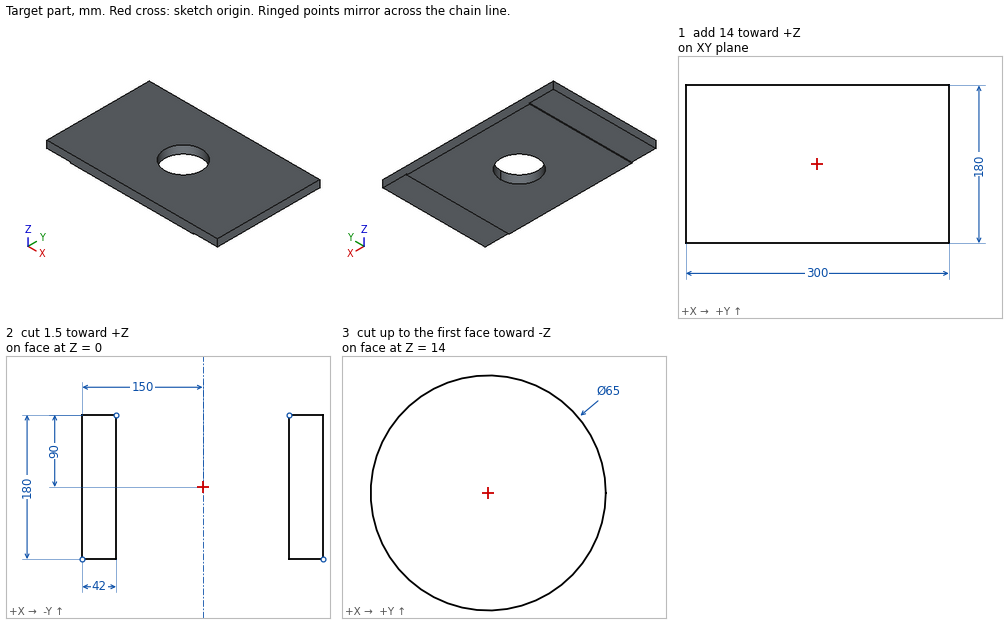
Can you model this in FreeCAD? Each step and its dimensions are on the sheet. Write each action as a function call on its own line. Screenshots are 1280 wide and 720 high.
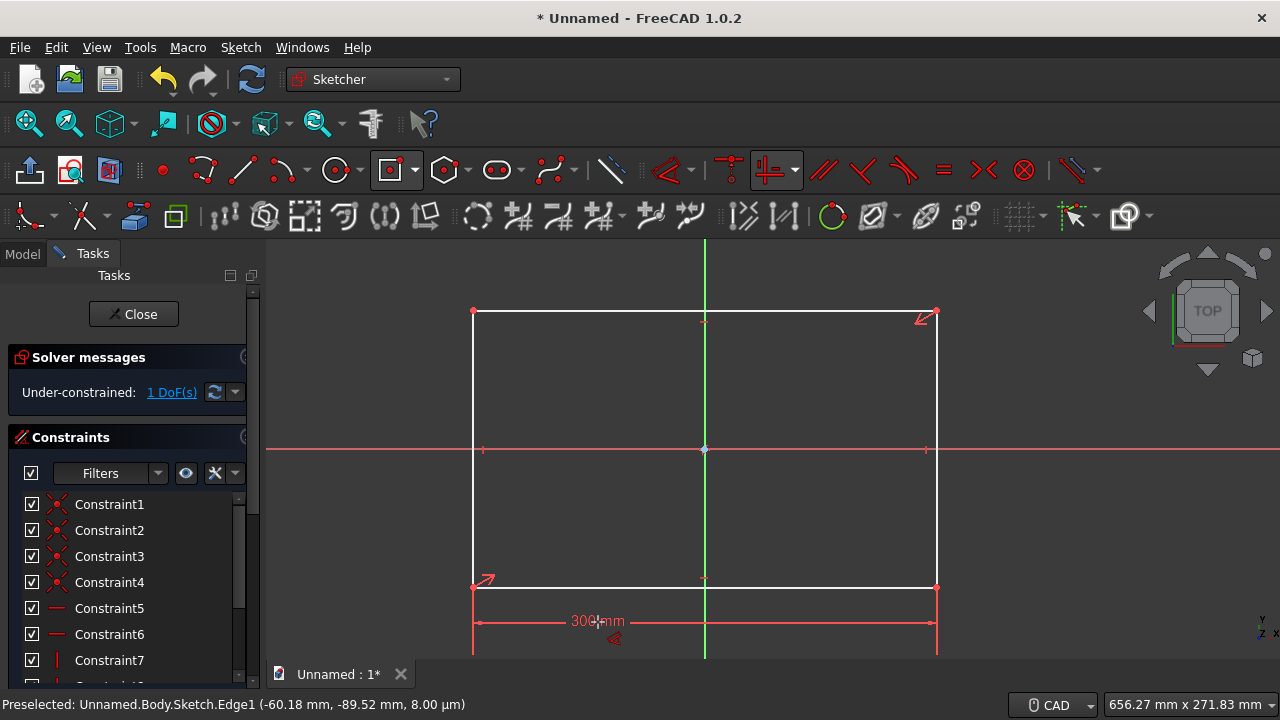
click(937, 505)
click(971, 386)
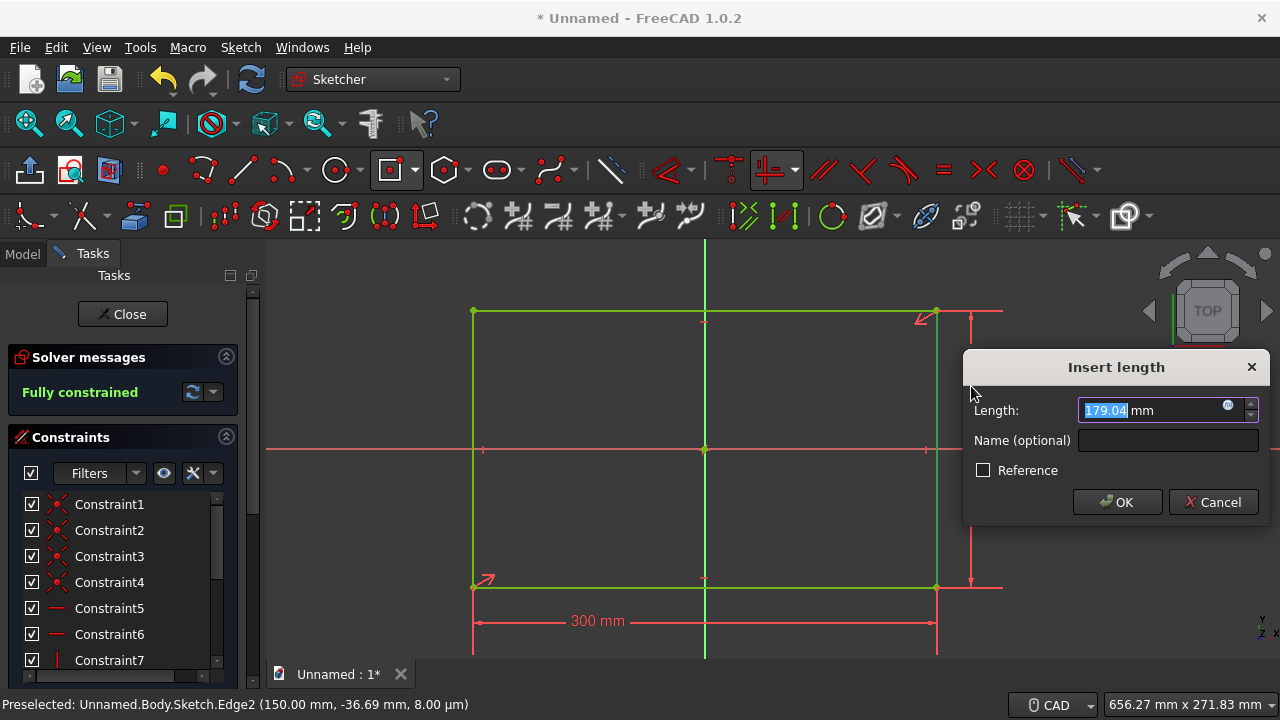
text(180)
key(Return)
key(Escape)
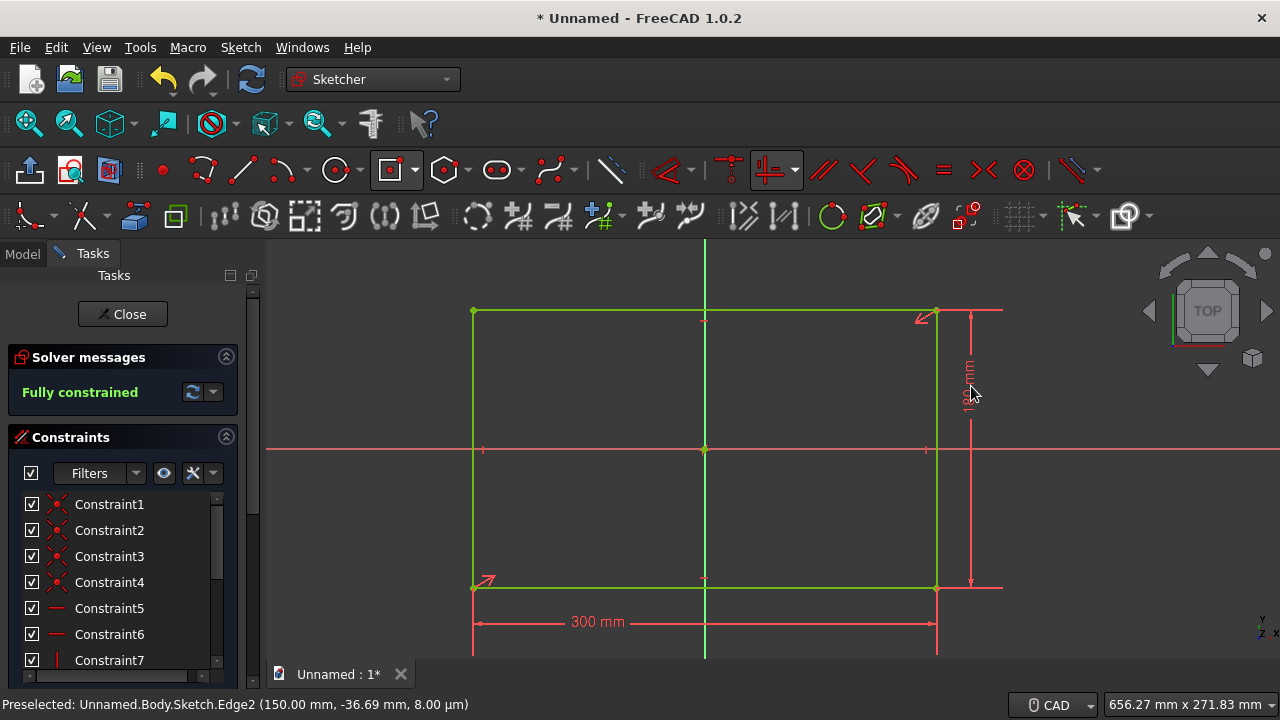
click(123, 314)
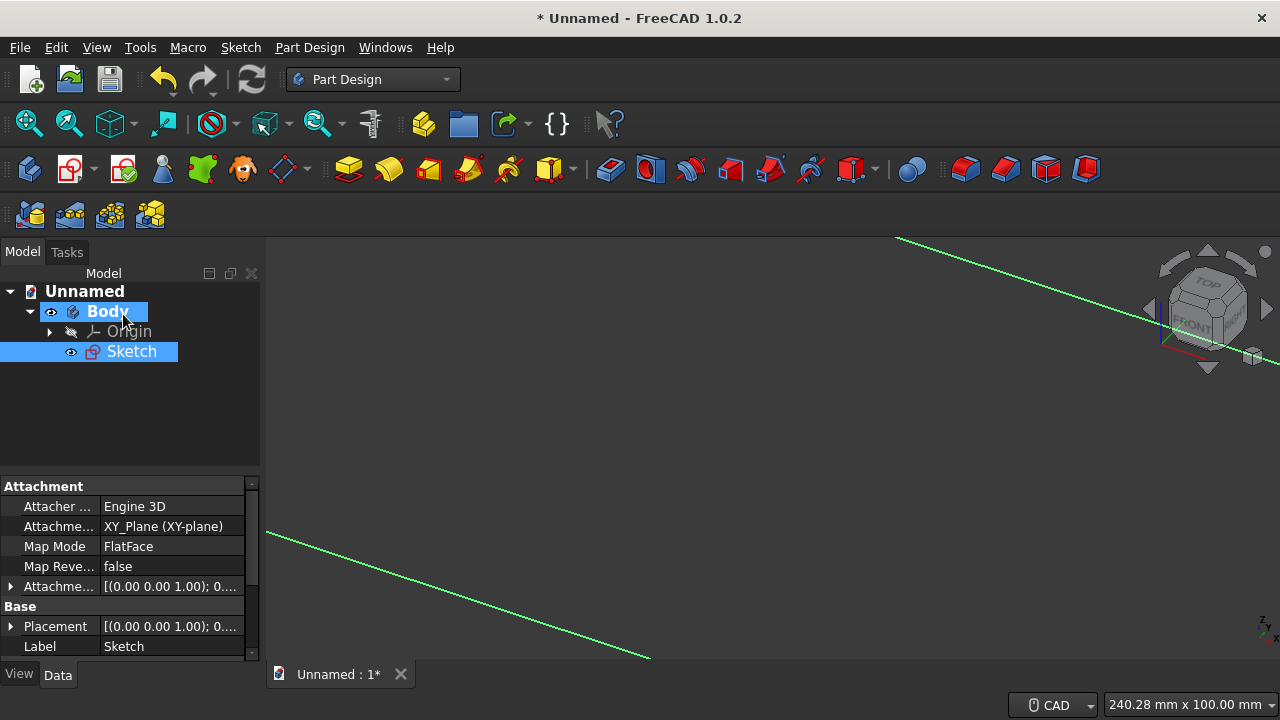
click(350, 170)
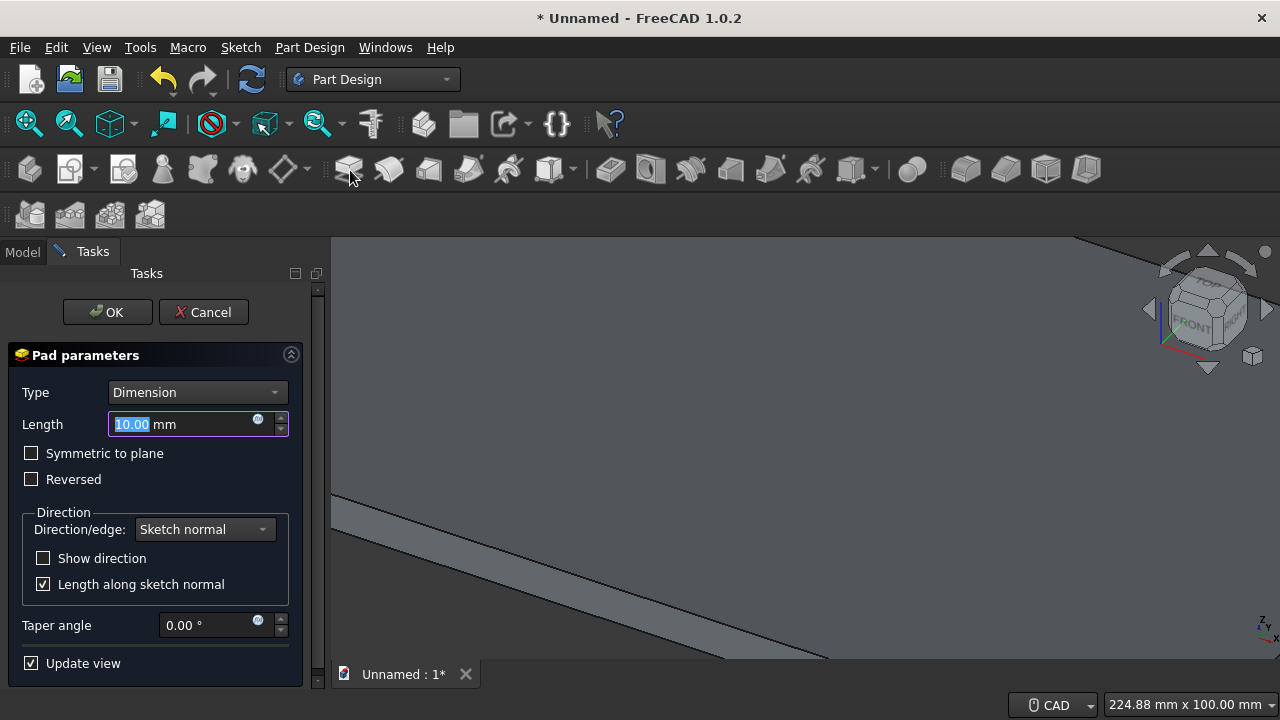
text(14)
key(Tab)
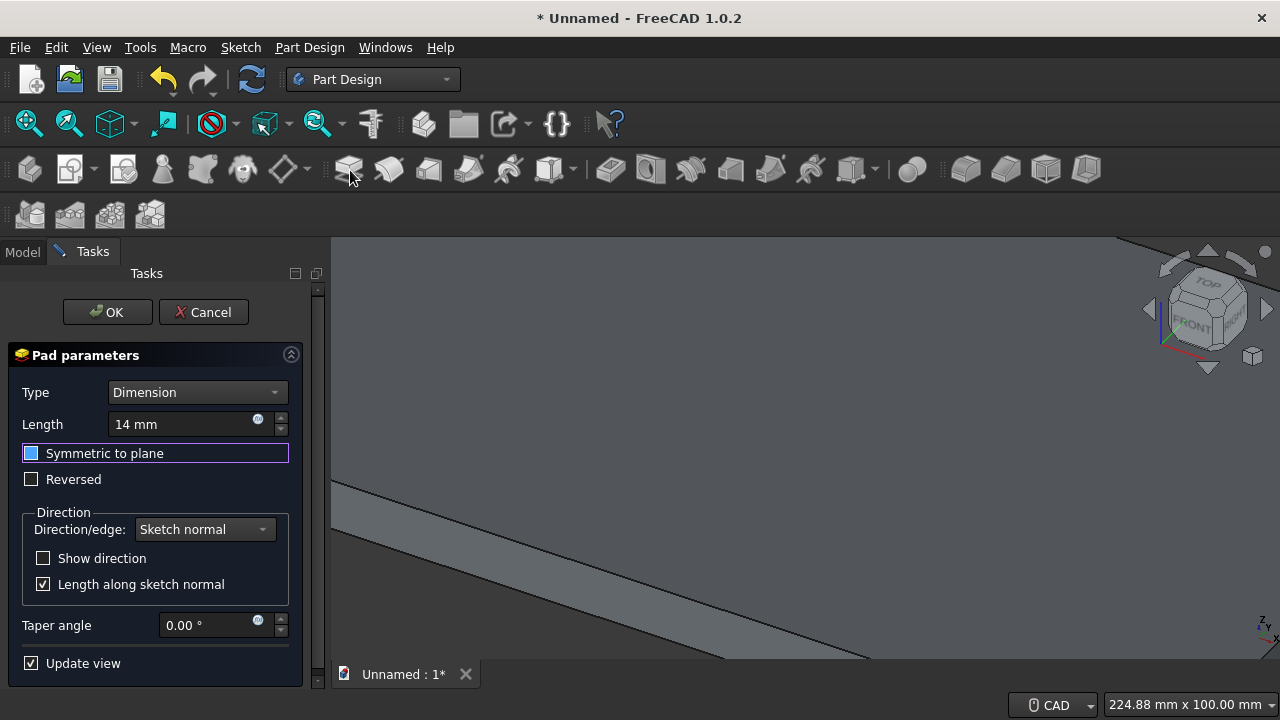
click(108, 312)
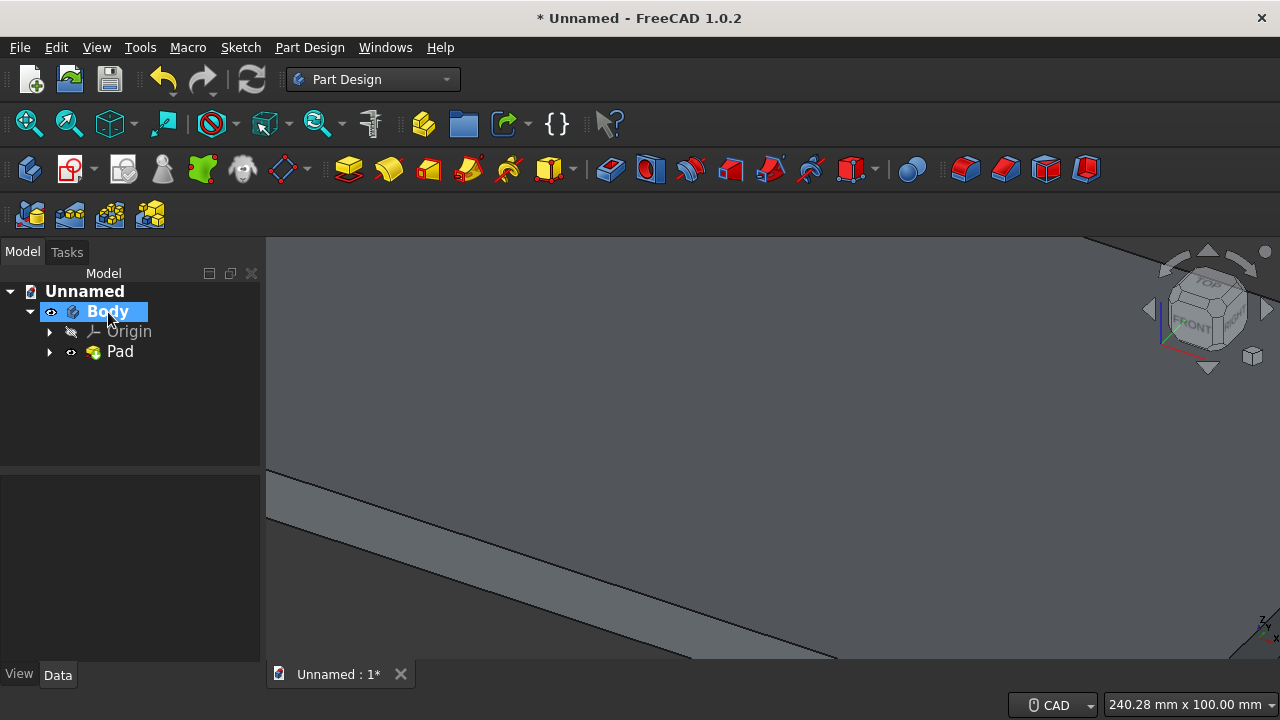
click(30, 124)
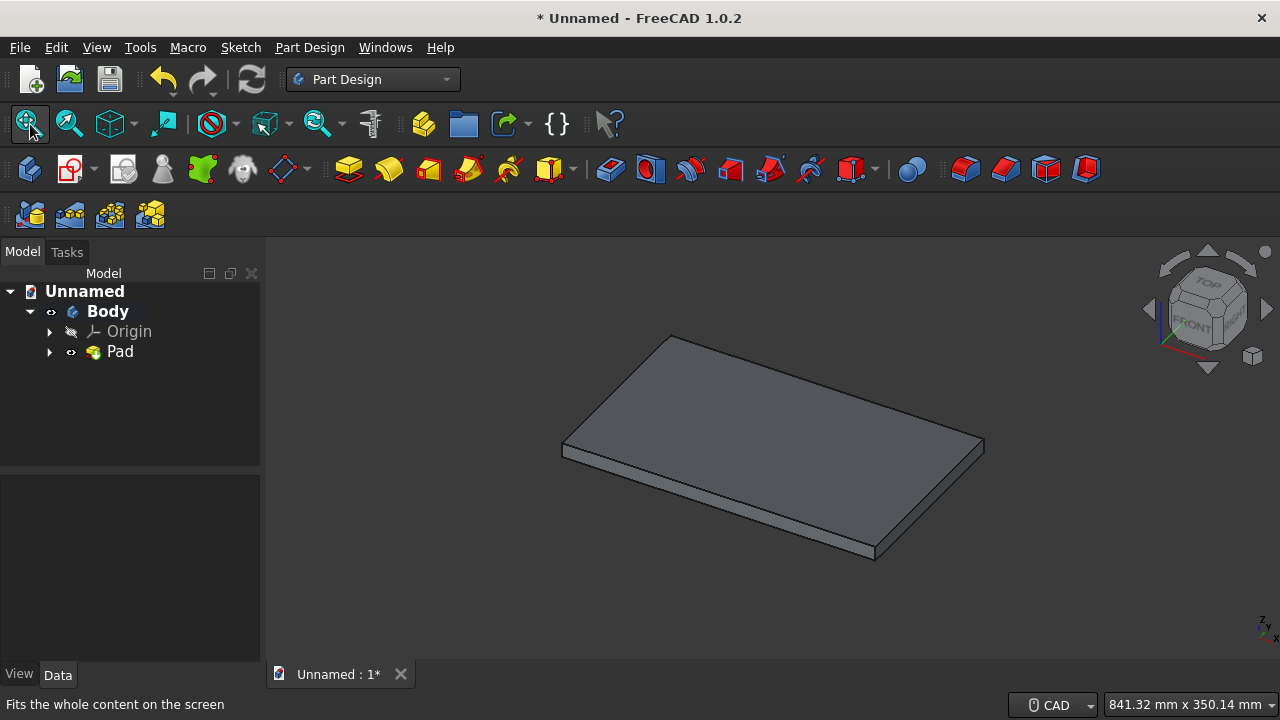
key(5)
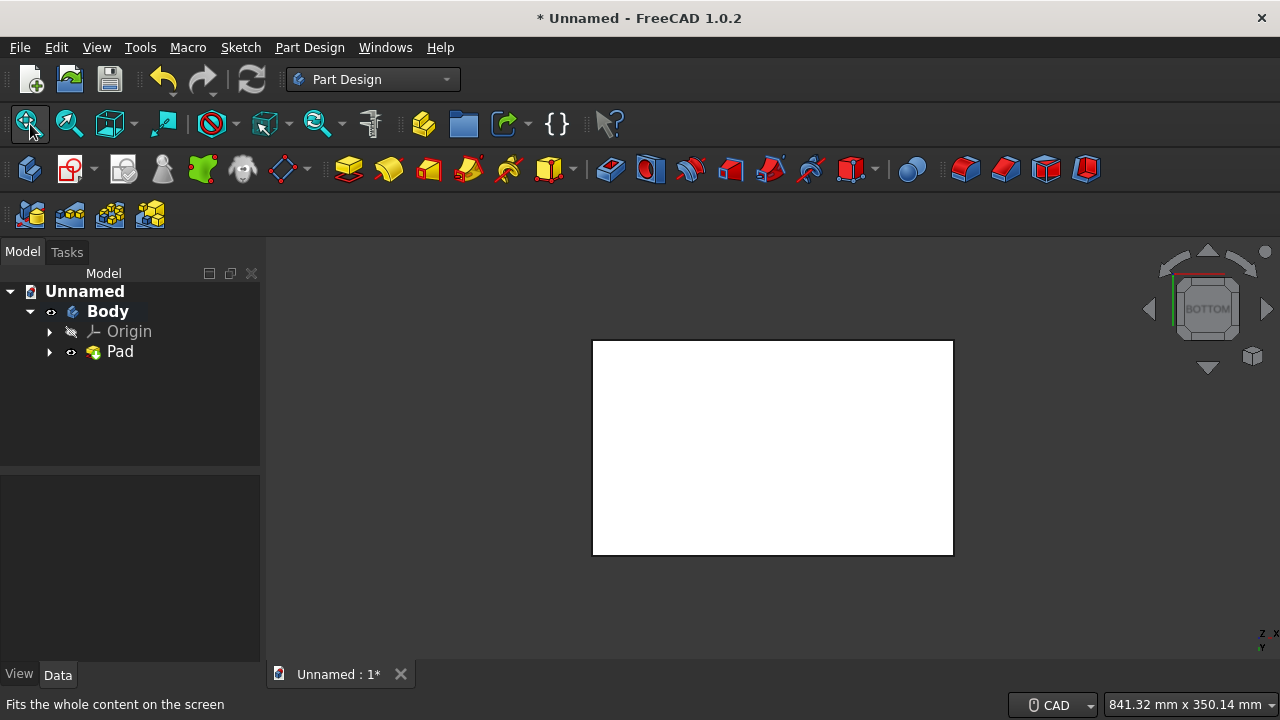
click(825, 447)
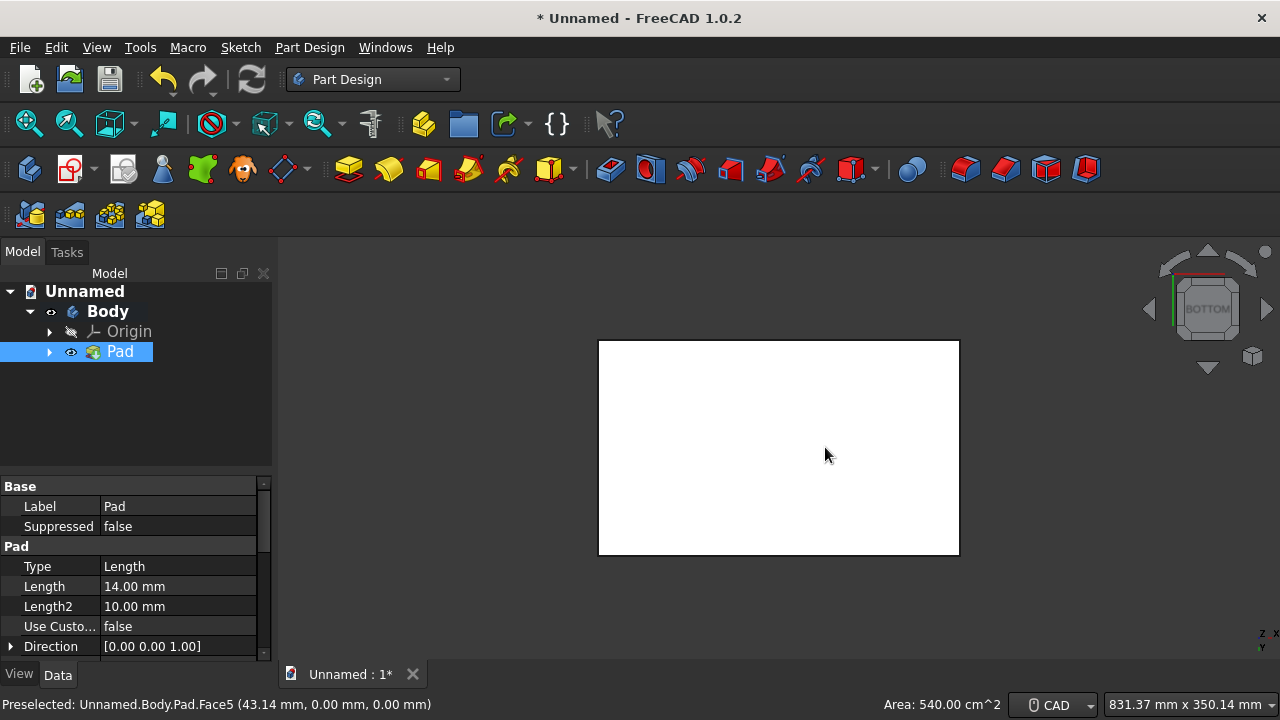
click(70, 170)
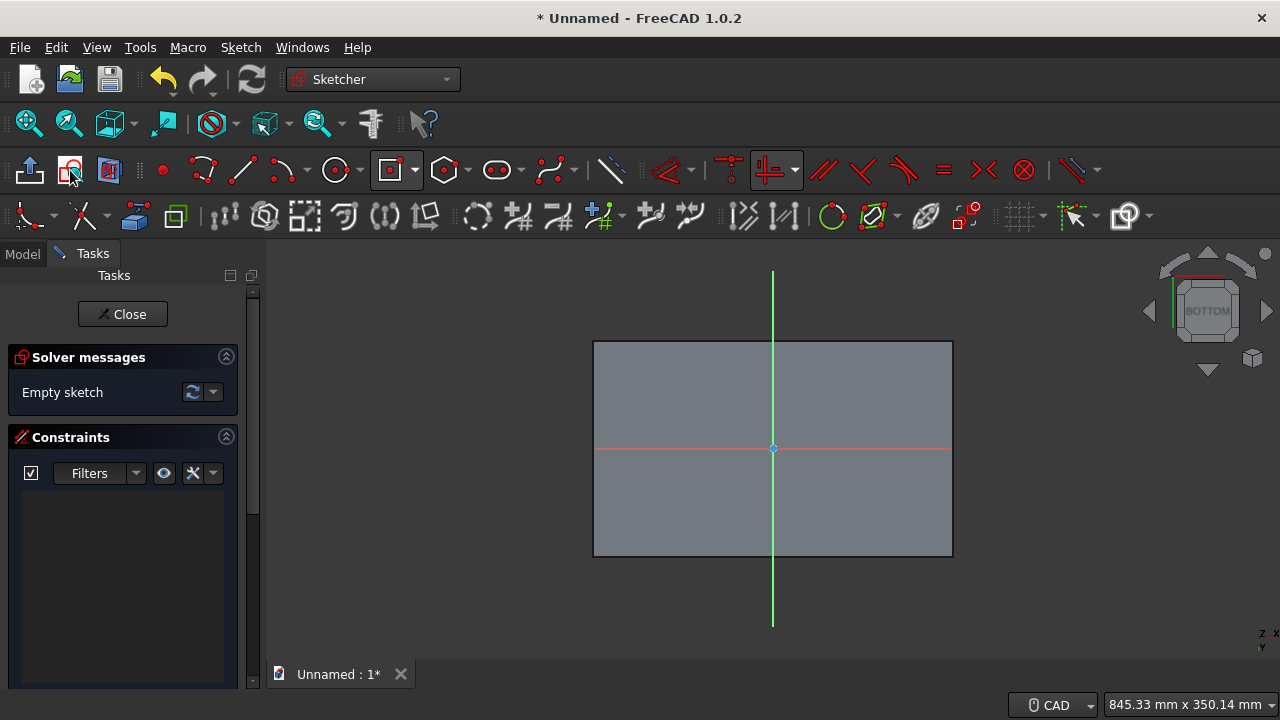
click(418, 170)